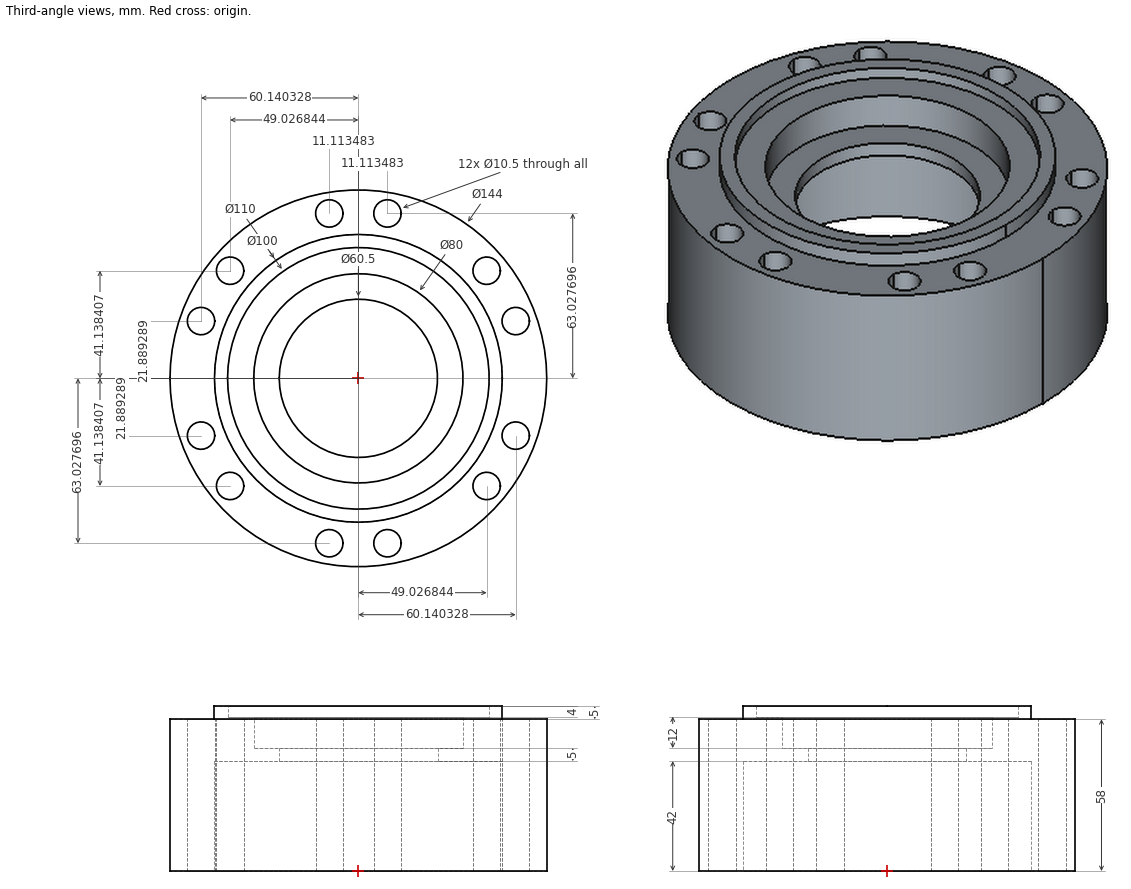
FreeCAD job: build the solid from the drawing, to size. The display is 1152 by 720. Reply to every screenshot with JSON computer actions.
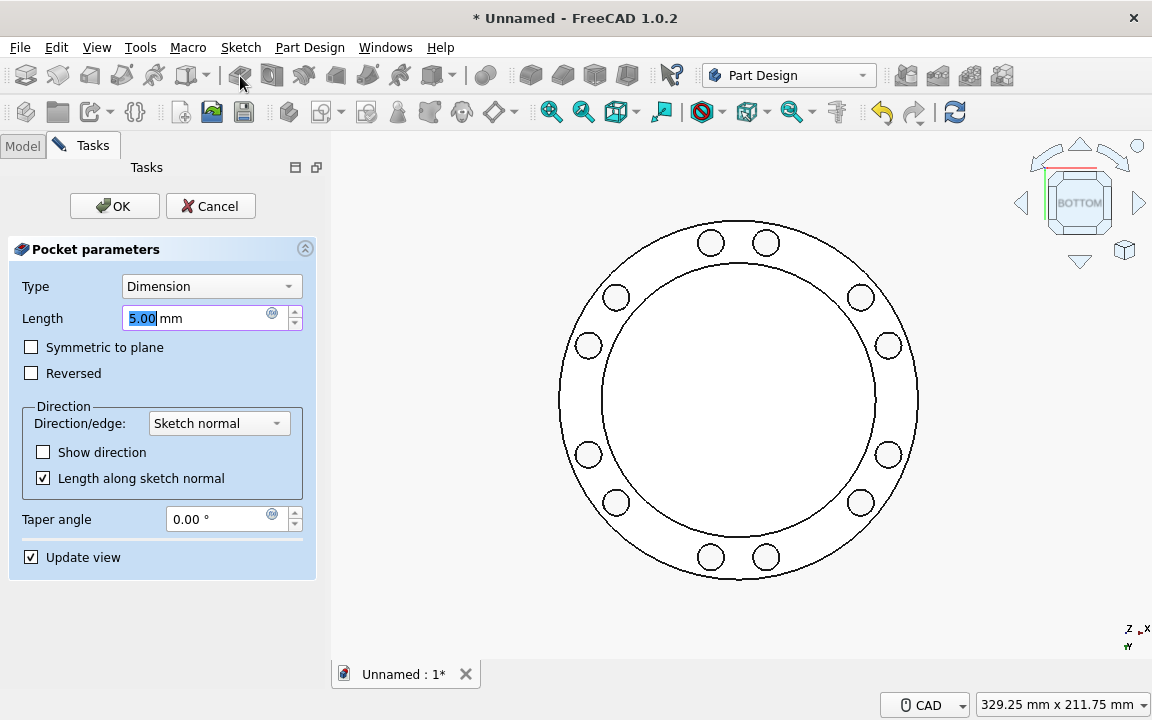
{"action": "type", "text": "42"}
{"action": "key", "text": "Tab"}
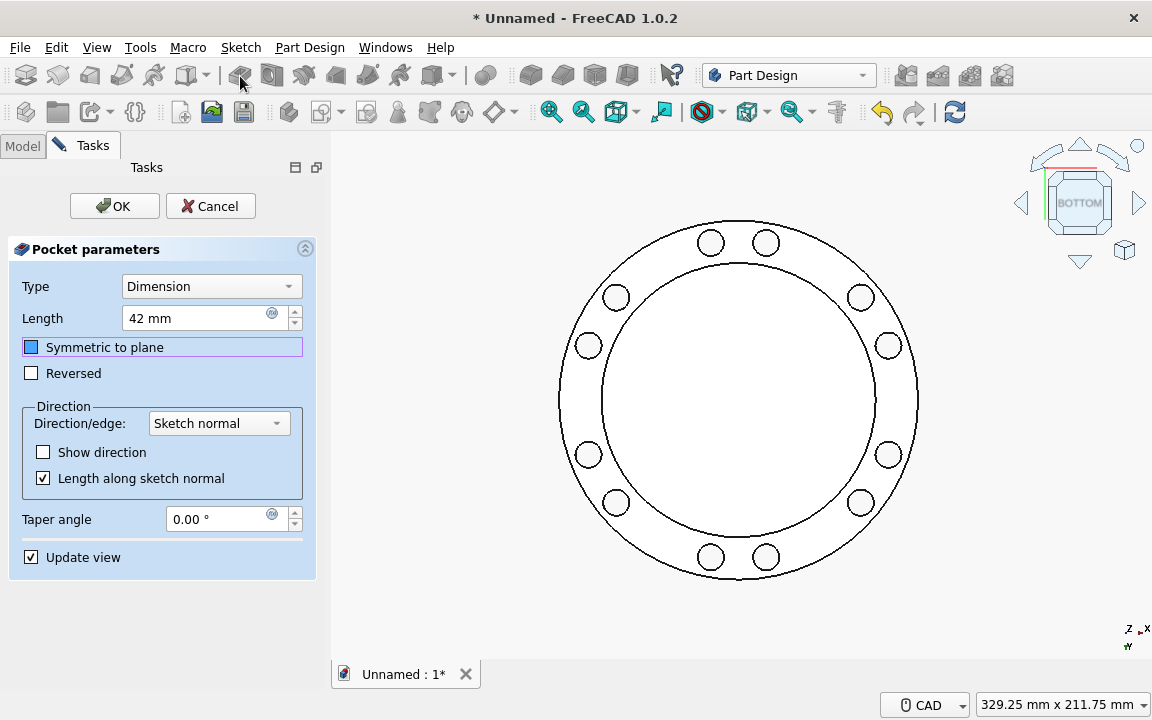
{"action": "left_click", "coordinate": [115, 206]}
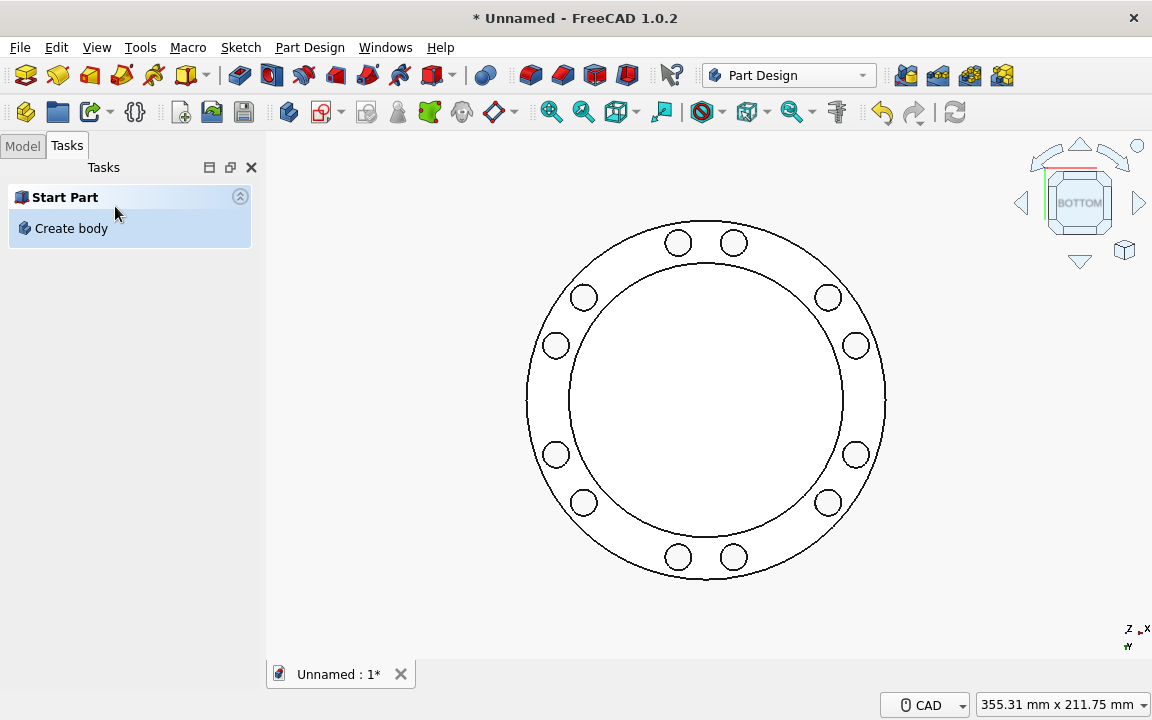
{"action": "left_click", "coordinate": [706, 399]}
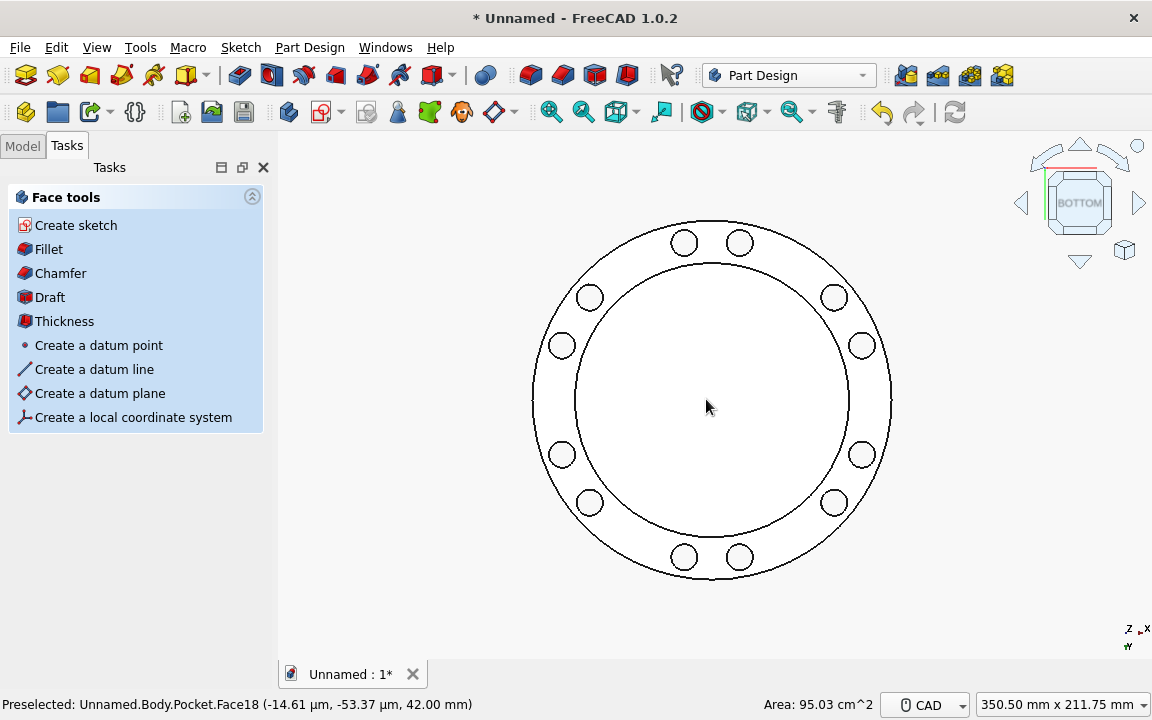
{"action": "left_click", "coordinate": [322, 112]}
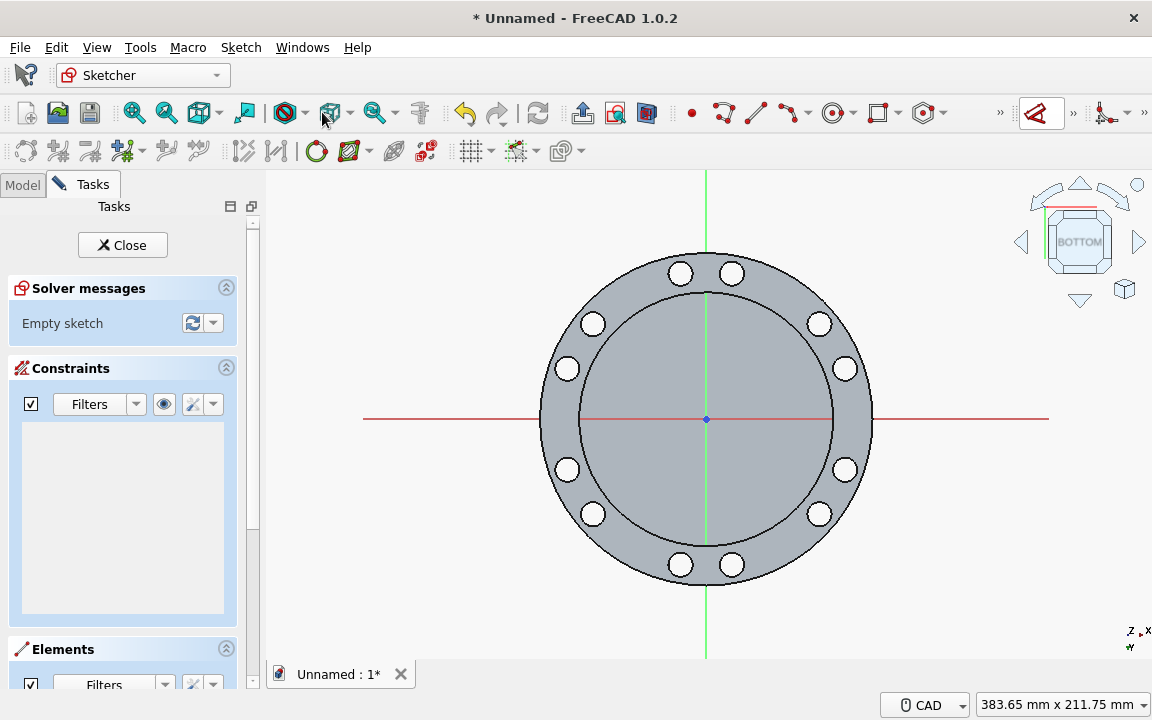
{"action": "key", "text": "q s"}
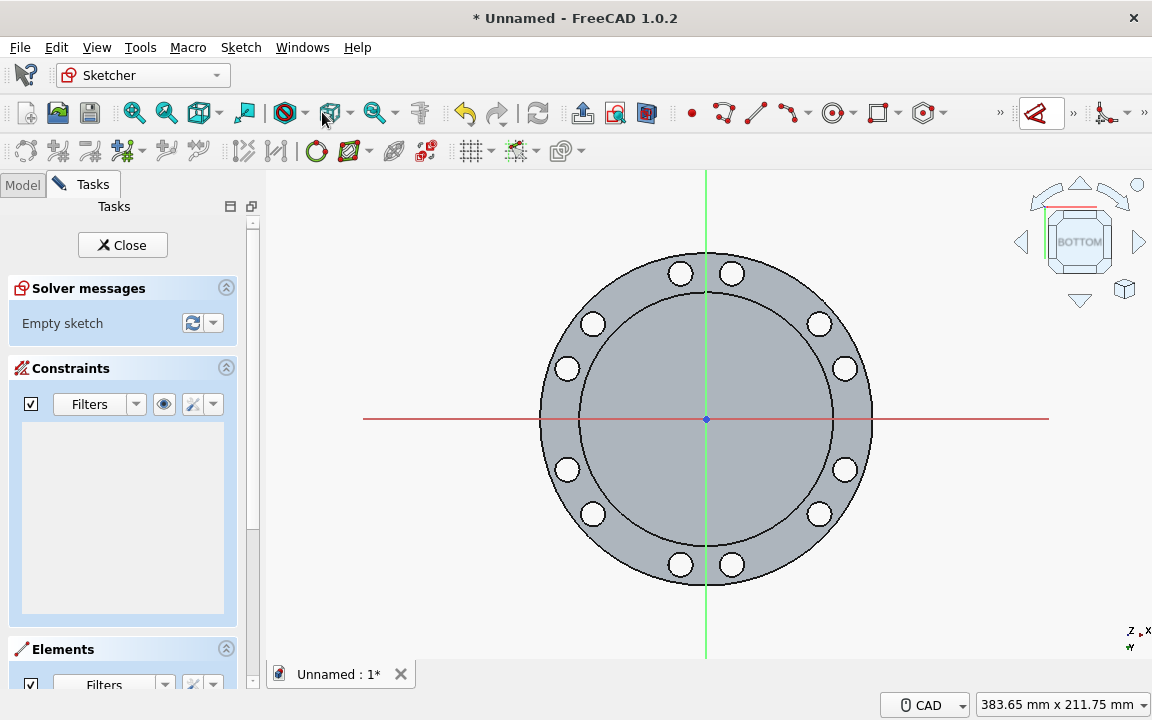
{"action": "scroll", "coordinate": [760, 423], "scroll_direction": "up", "scroll_amount": 4}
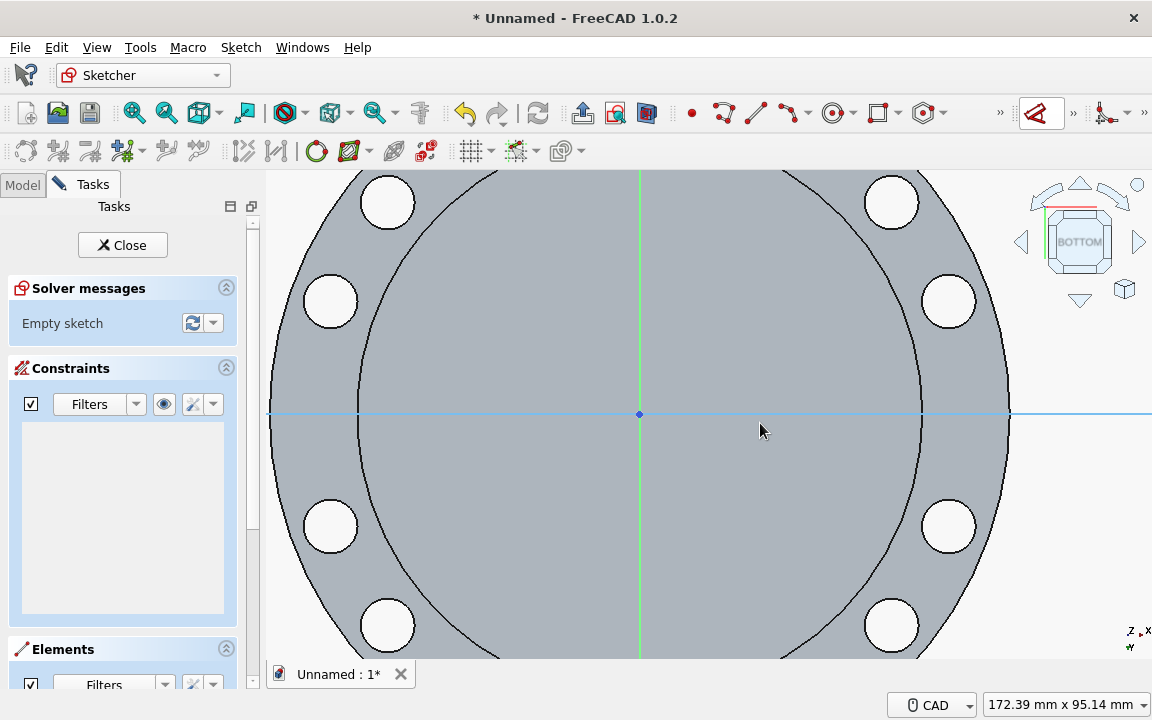
{"action": "key", "text": "g c"}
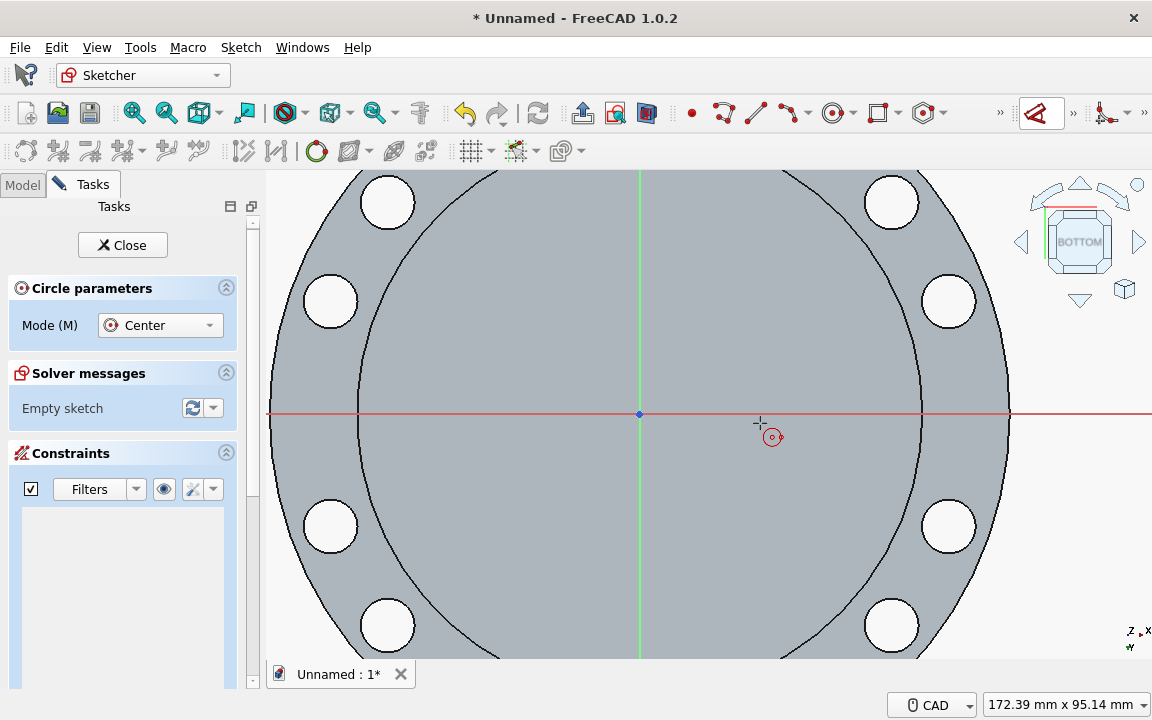
{"action": "left_click", "coordinate": [640, 414]}
{"action": "left_click", "coordinate": [750, 304]}
{"action": "key", "text": "Escape"}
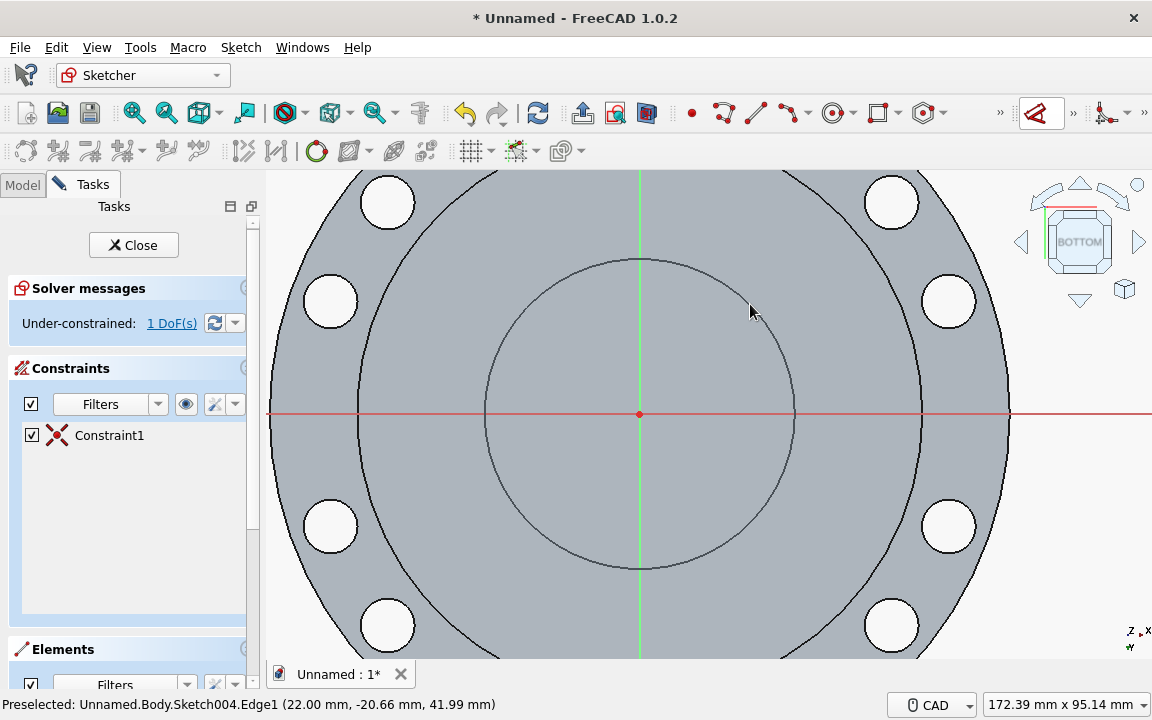
{"action": "key", "text": "d"}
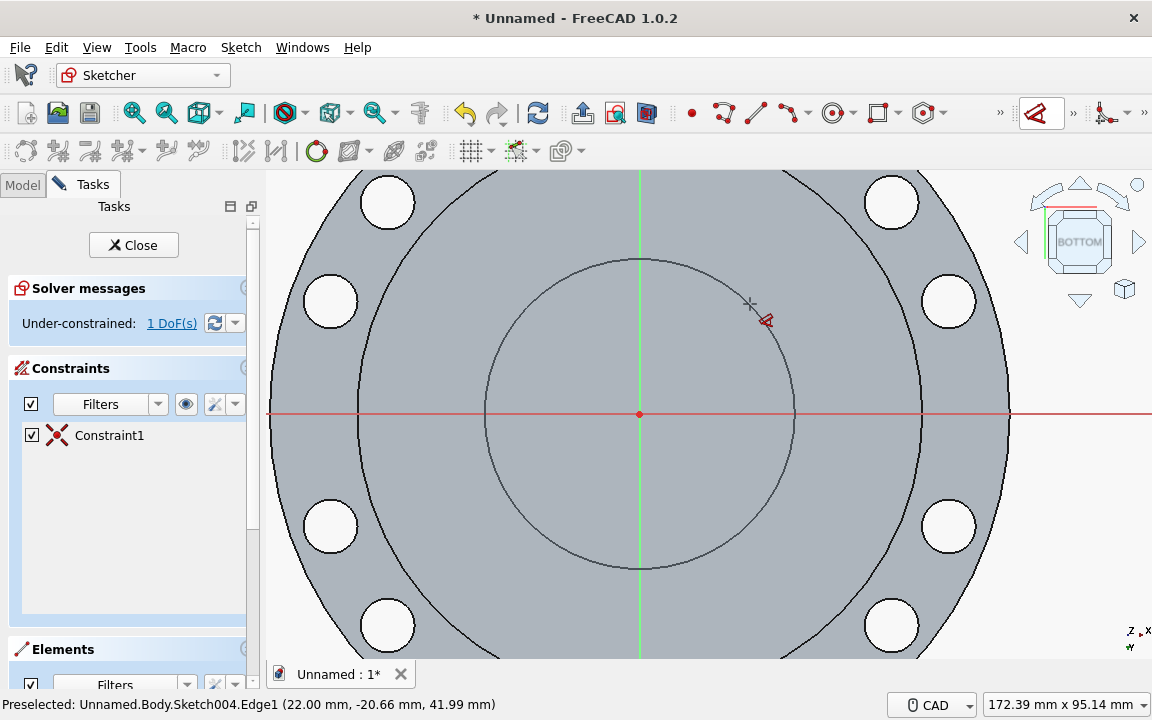
{"action": "left_click", "coordinate": [749, 304]}
{"action": "left_click", "coordinate": [772, 281]}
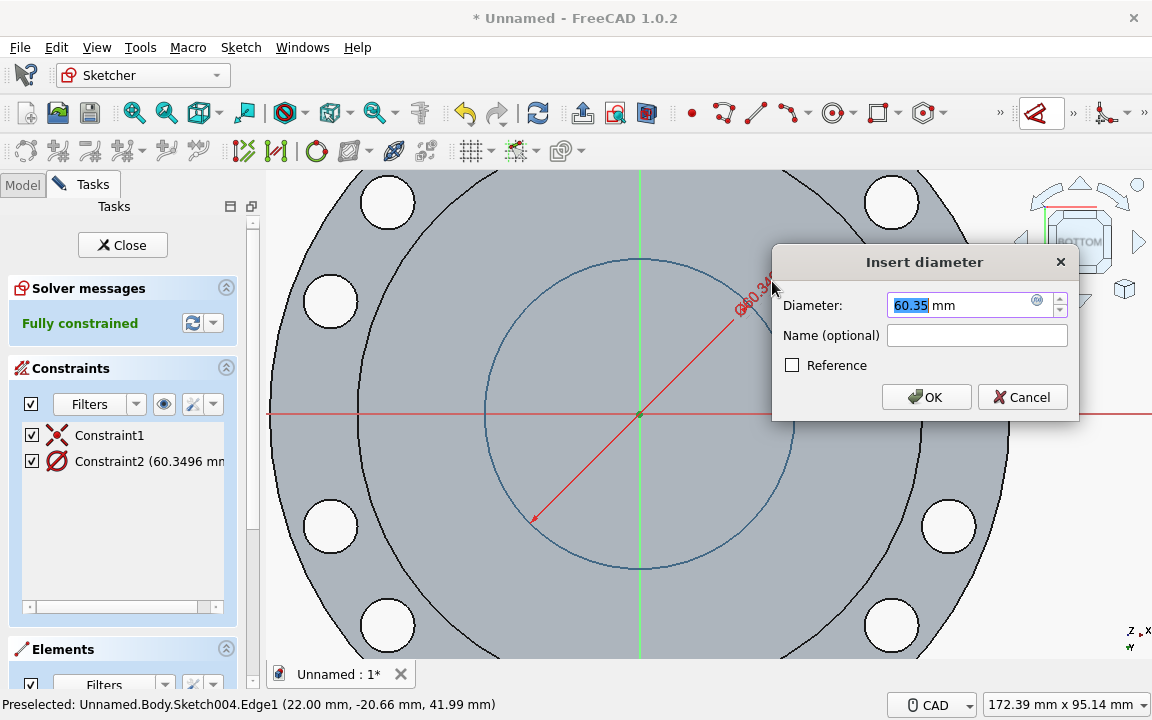
{"action": "type", "text": "60.5"}
{"action": "key", "text": "Return"}
{"action": "key", "text": "Escape"}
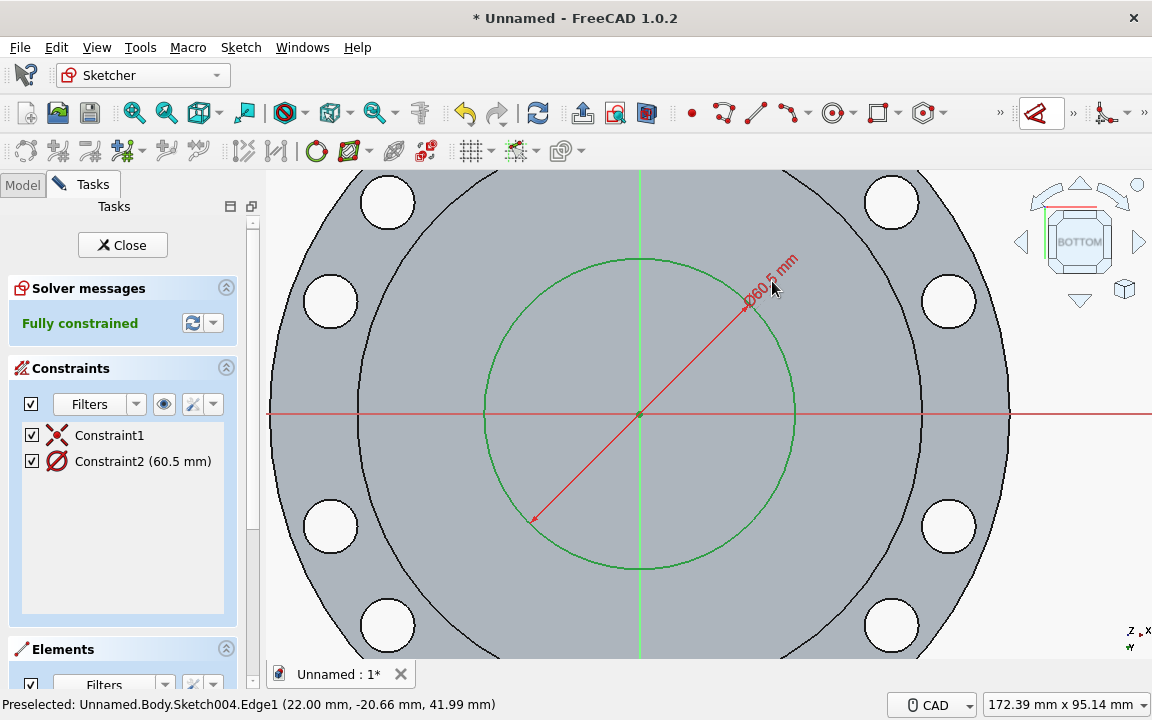
{"action": "left_click", "coordinate": [123, 245]}